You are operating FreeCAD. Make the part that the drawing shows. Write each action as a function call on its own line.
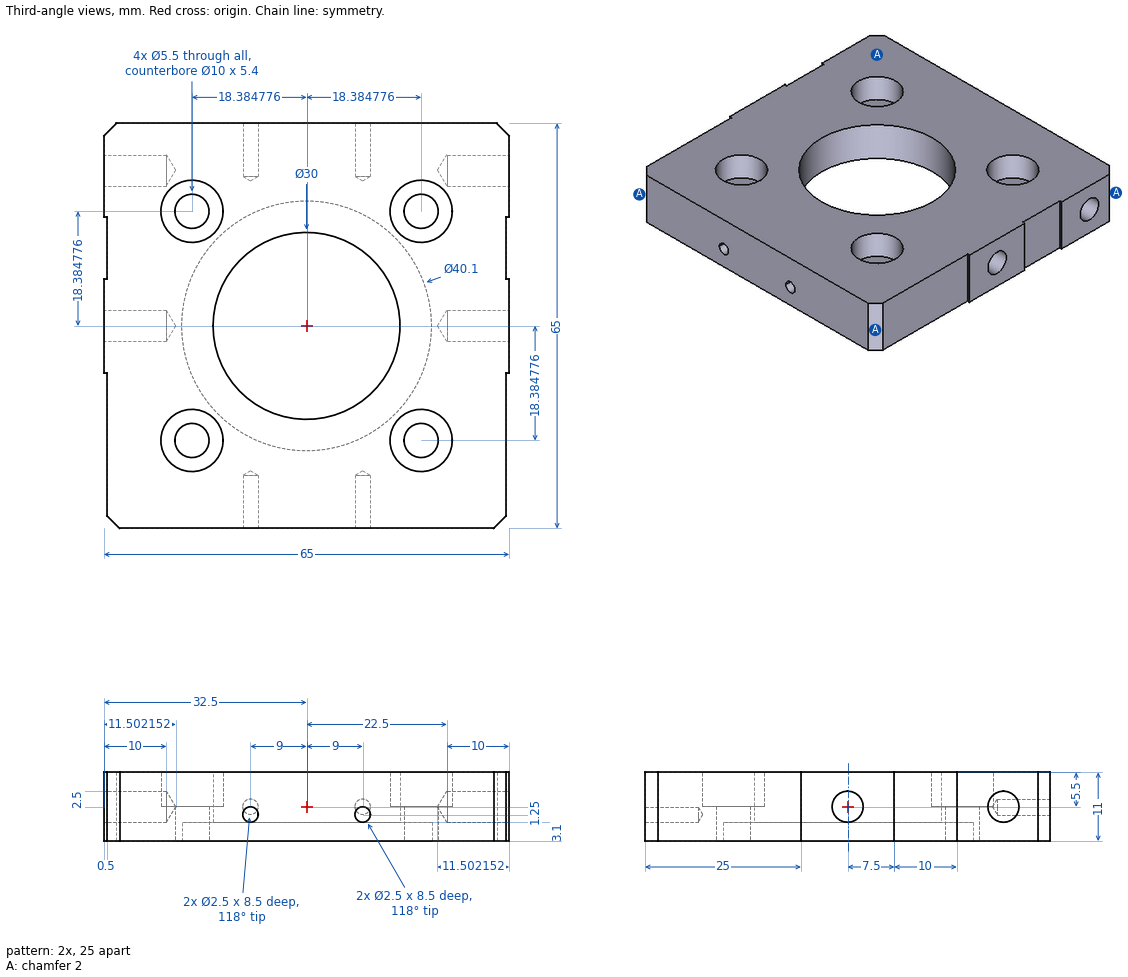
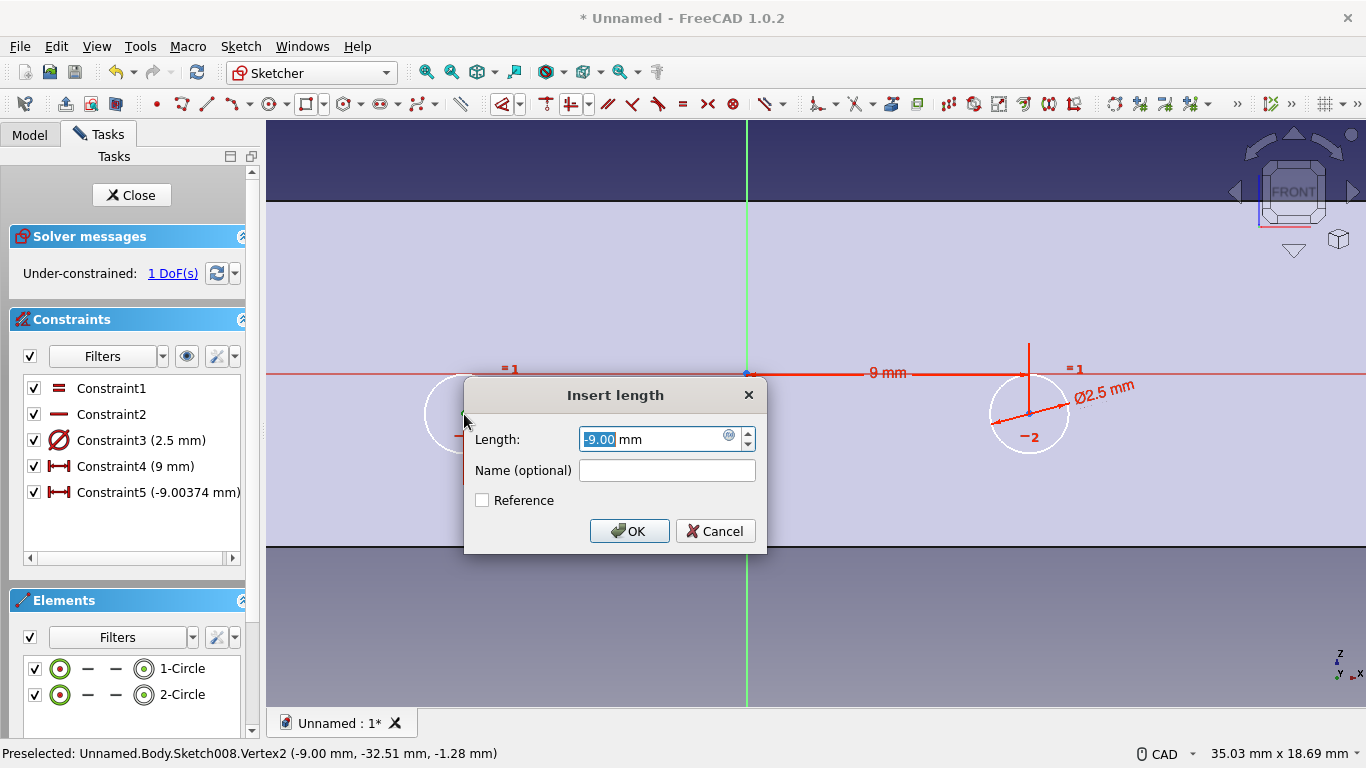
text(-9)
key(Return)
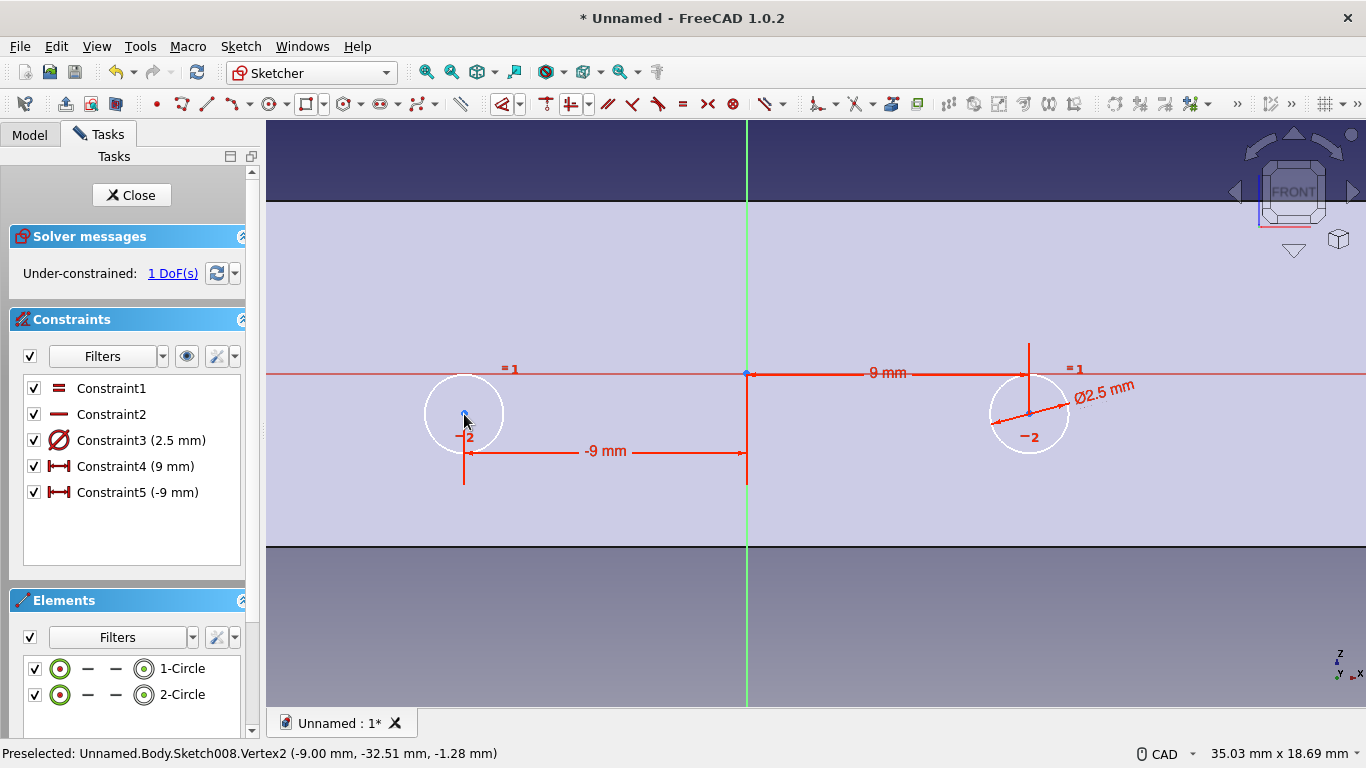
click(1029, 414)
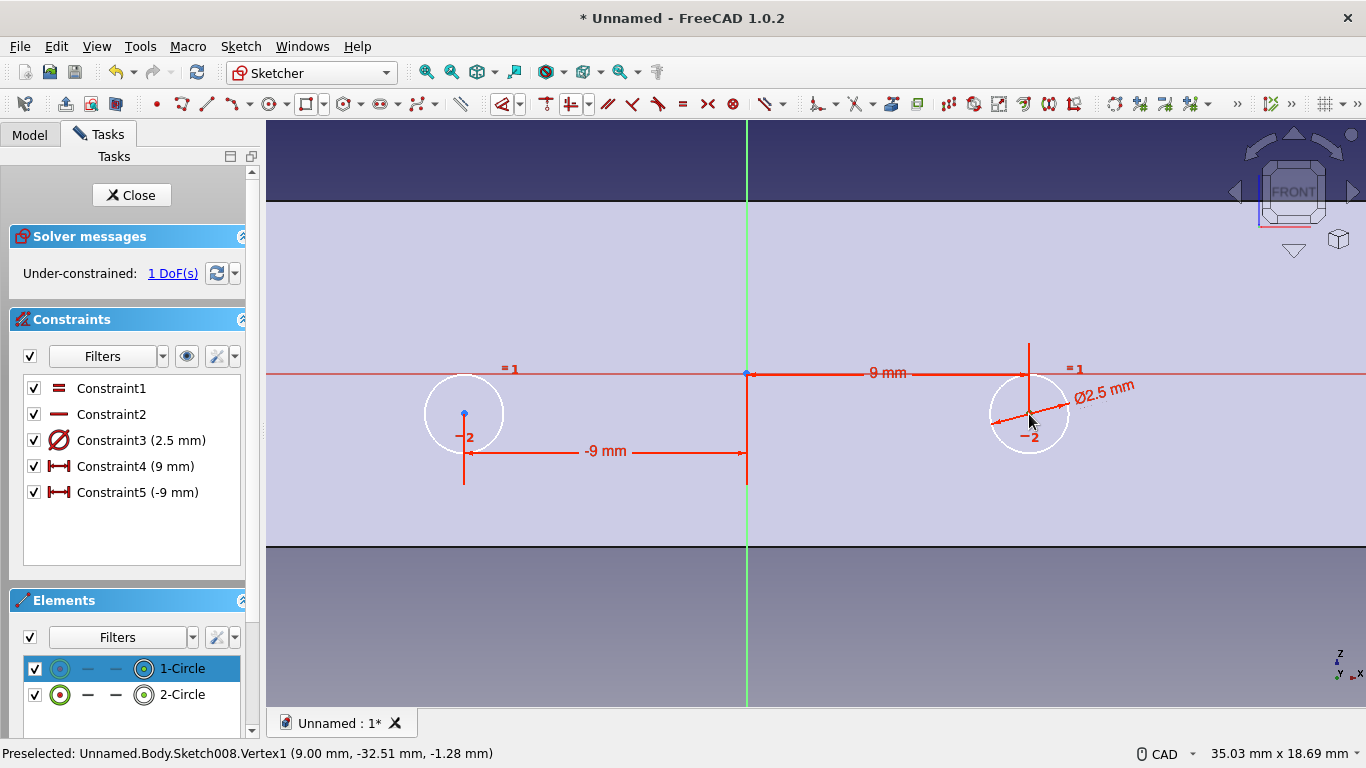
click(520, 104)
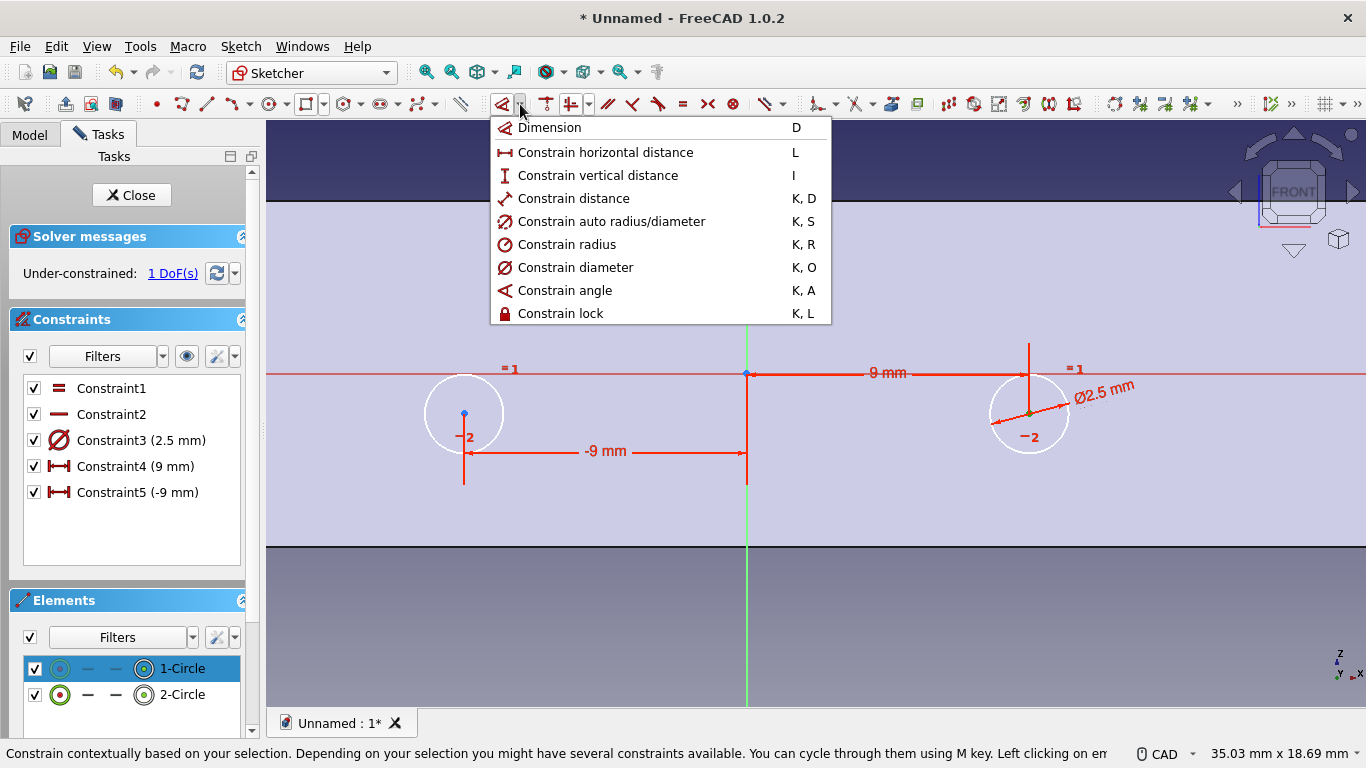
click(661, 176)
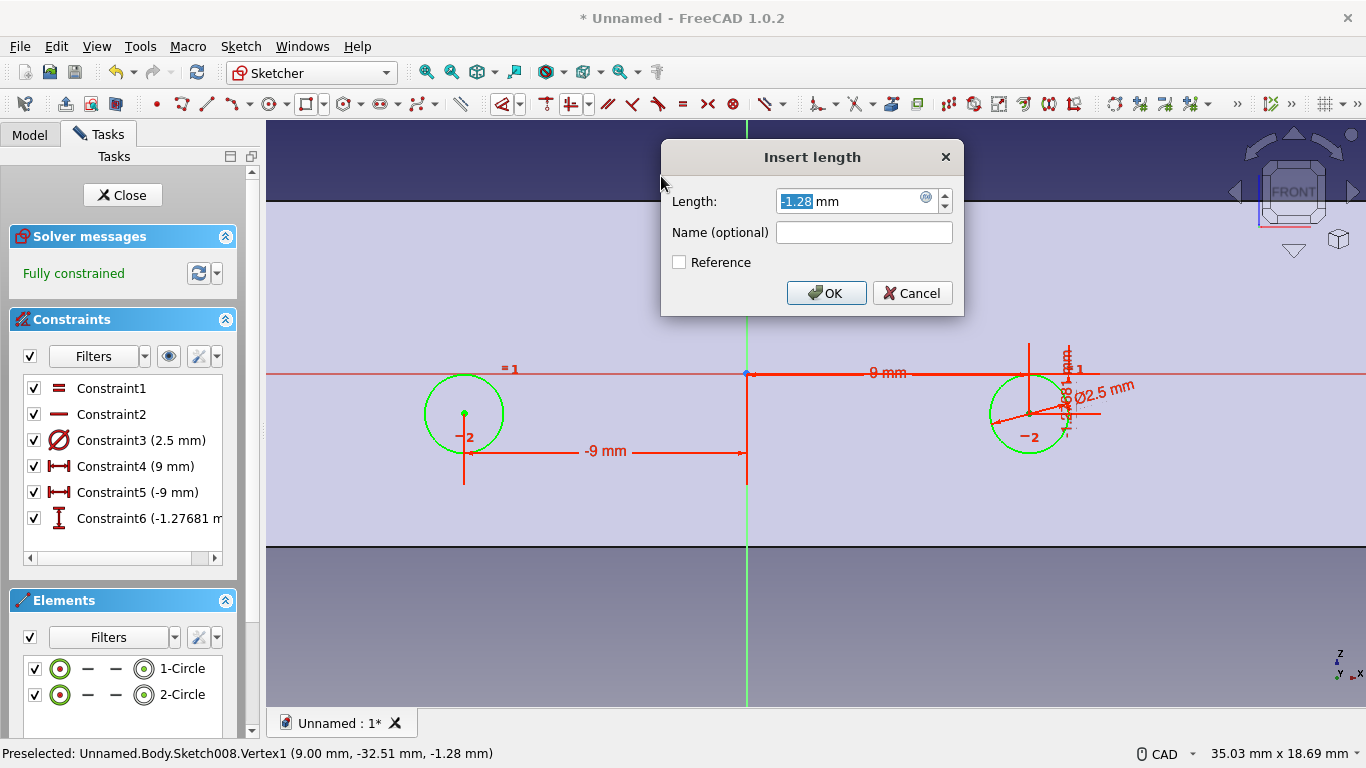
text(-1.25)
key(Return)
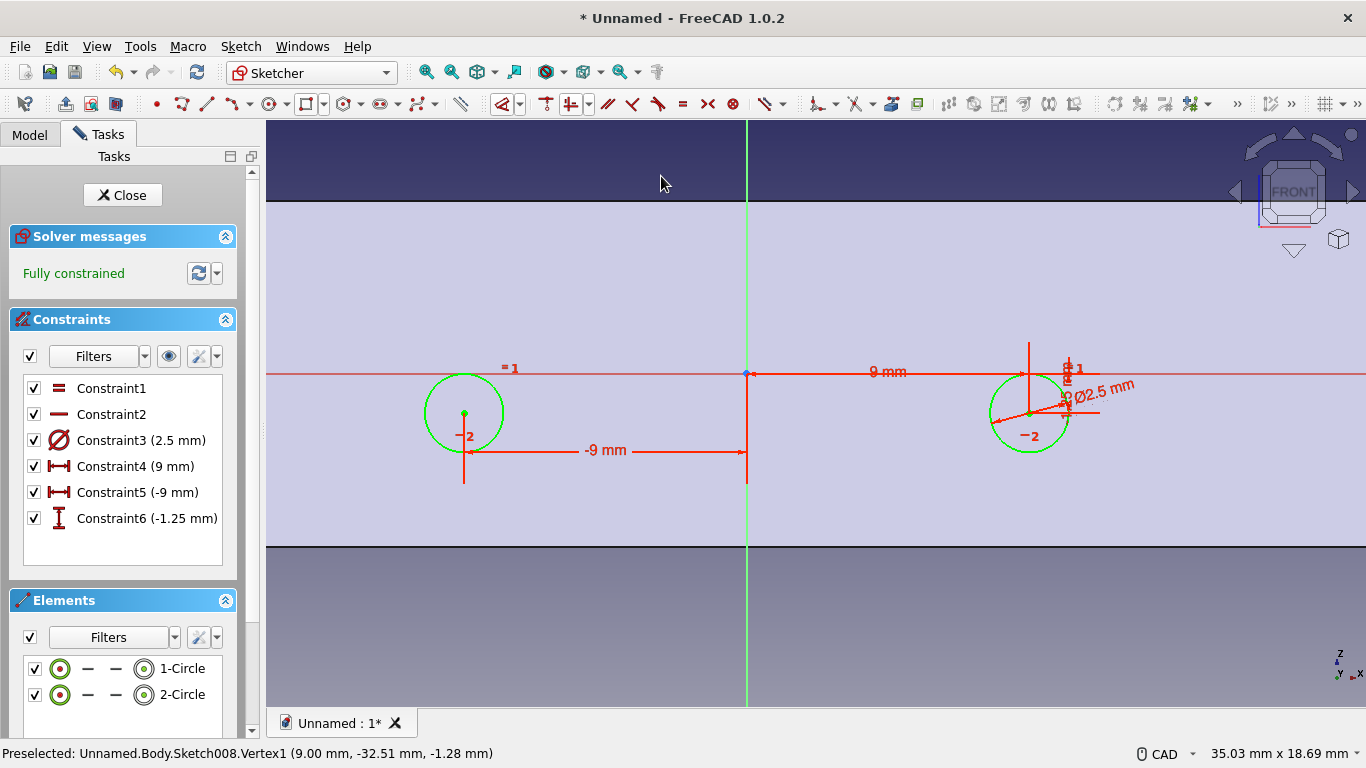
click(123, 195)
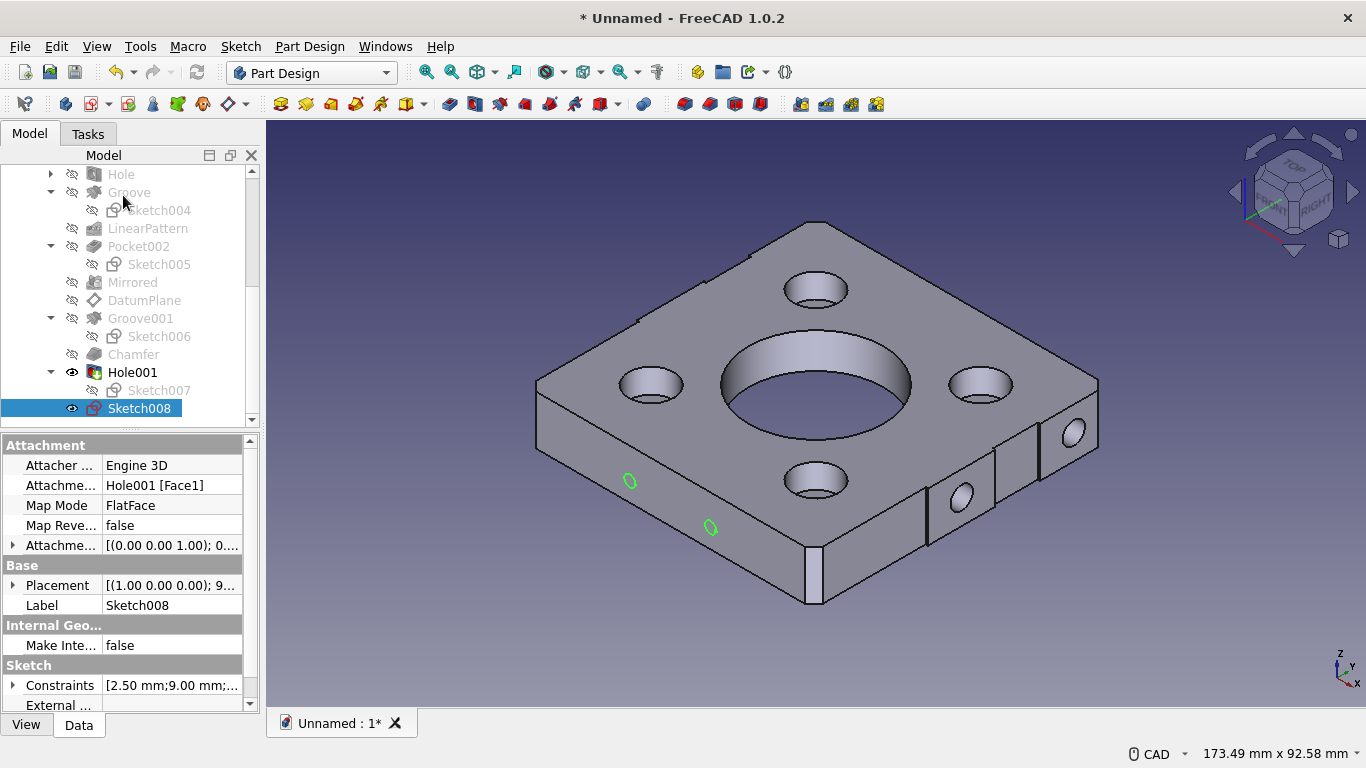
click(475, 104)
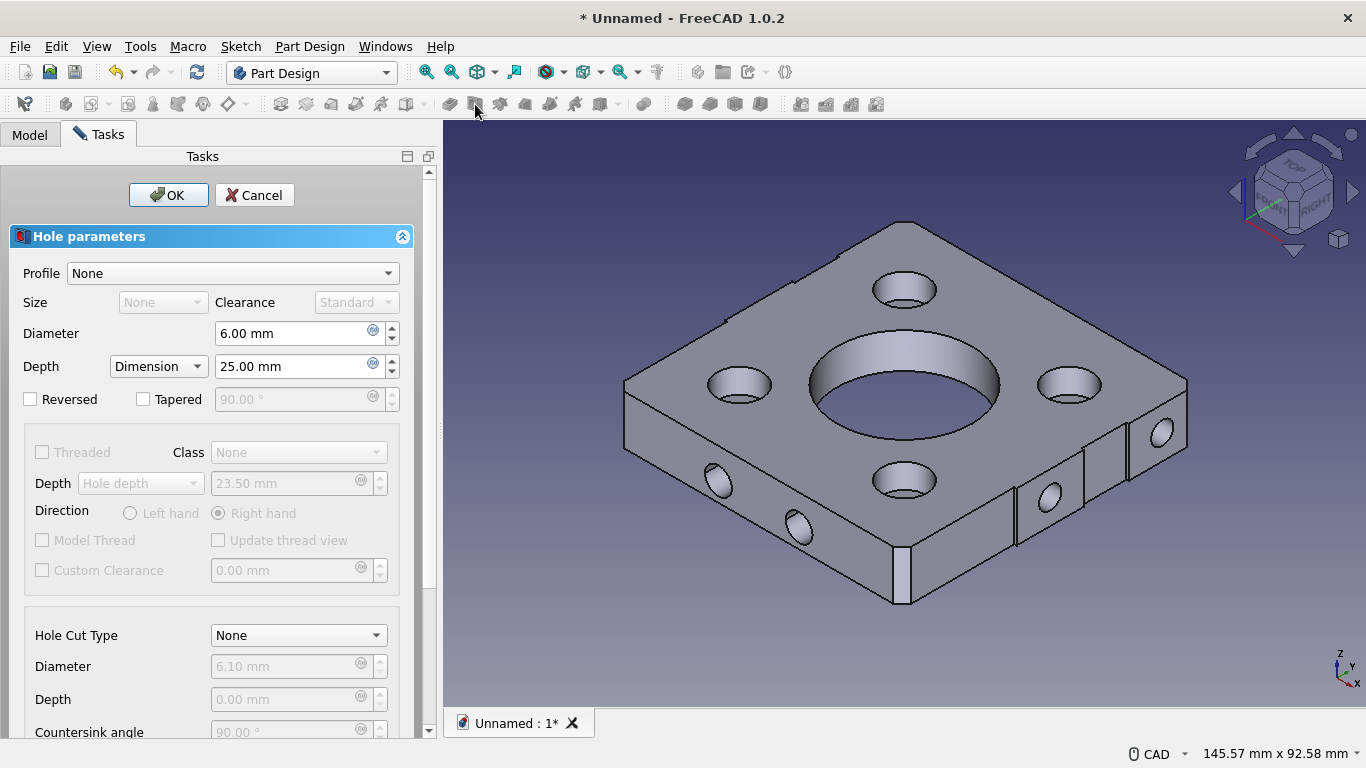
triple_click(300, 334)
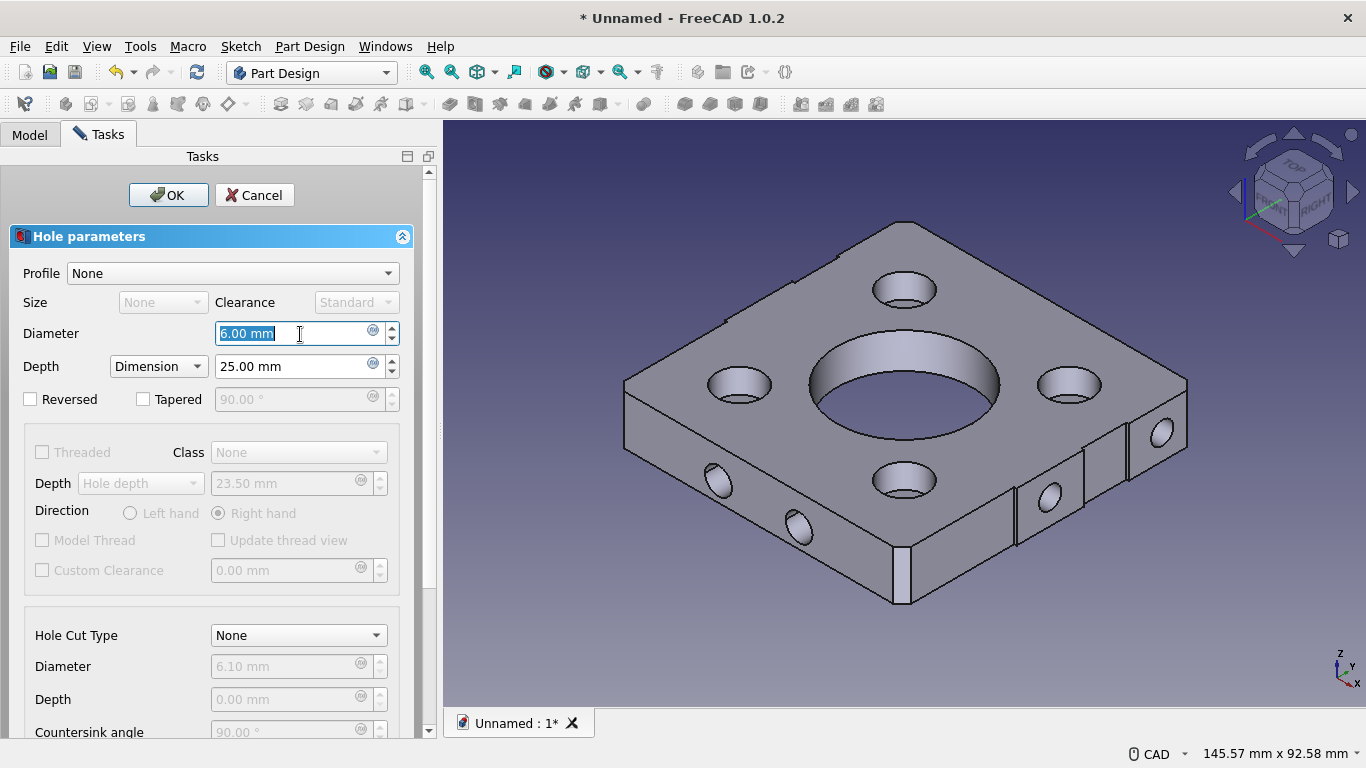
text(2.5)
key(Tab)